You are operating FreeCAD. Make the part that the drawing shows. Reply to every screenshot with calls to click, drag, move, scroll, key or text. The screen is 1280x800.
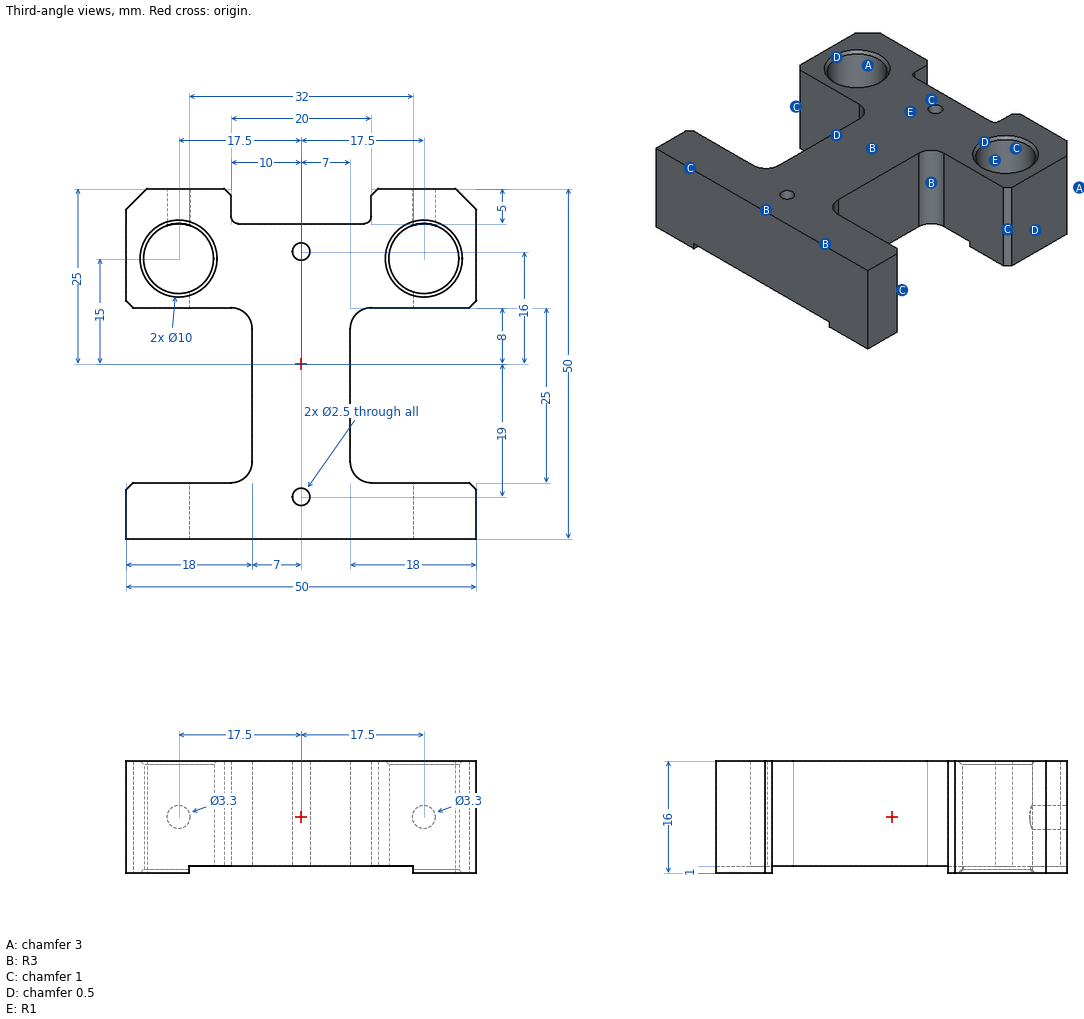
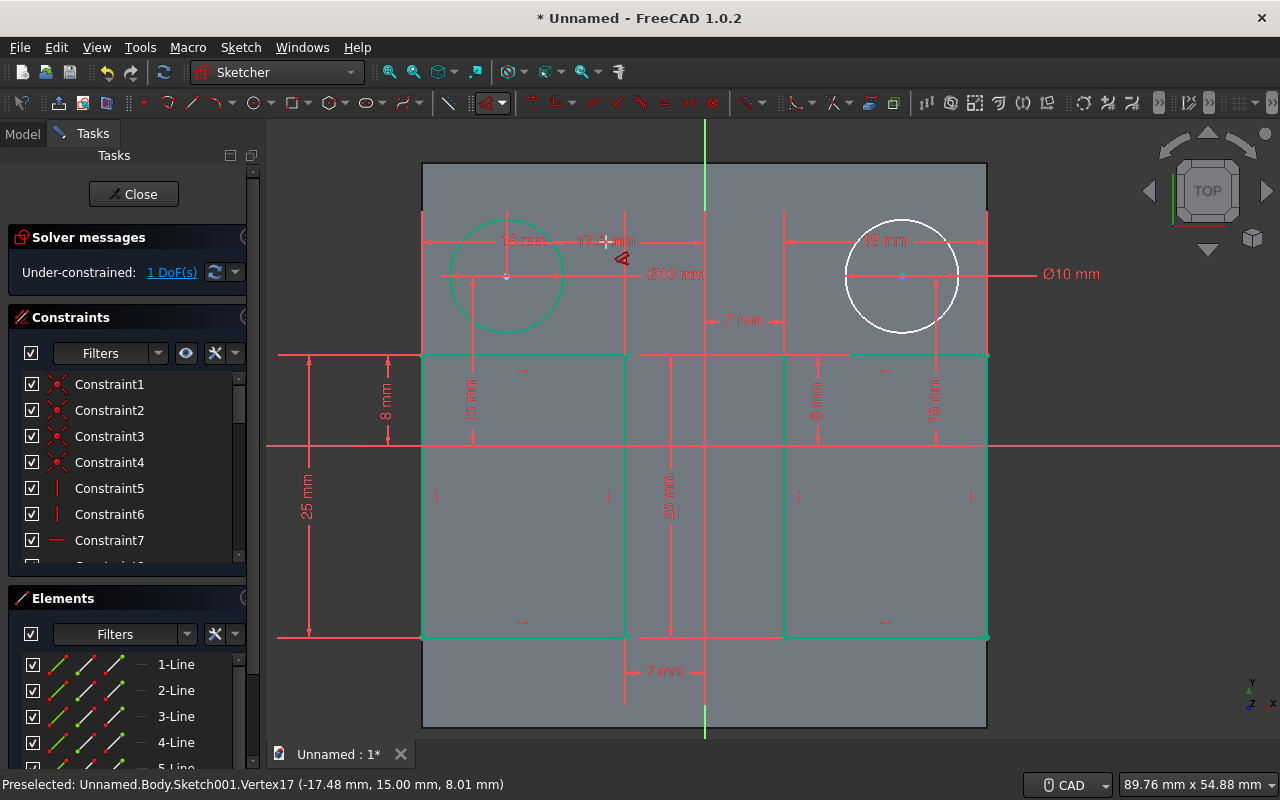
click(902, 276)
click(803, 242)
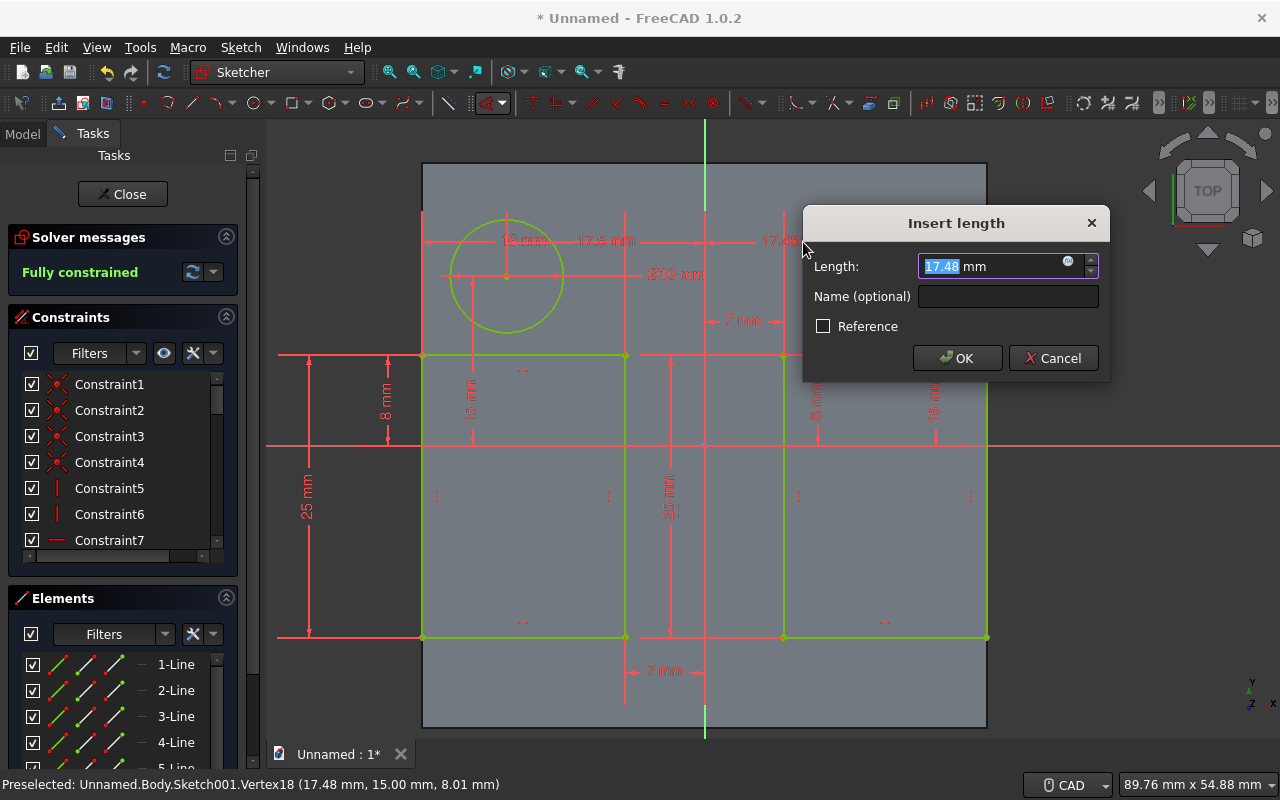
text(17.5)
key(Return)
key(Escape)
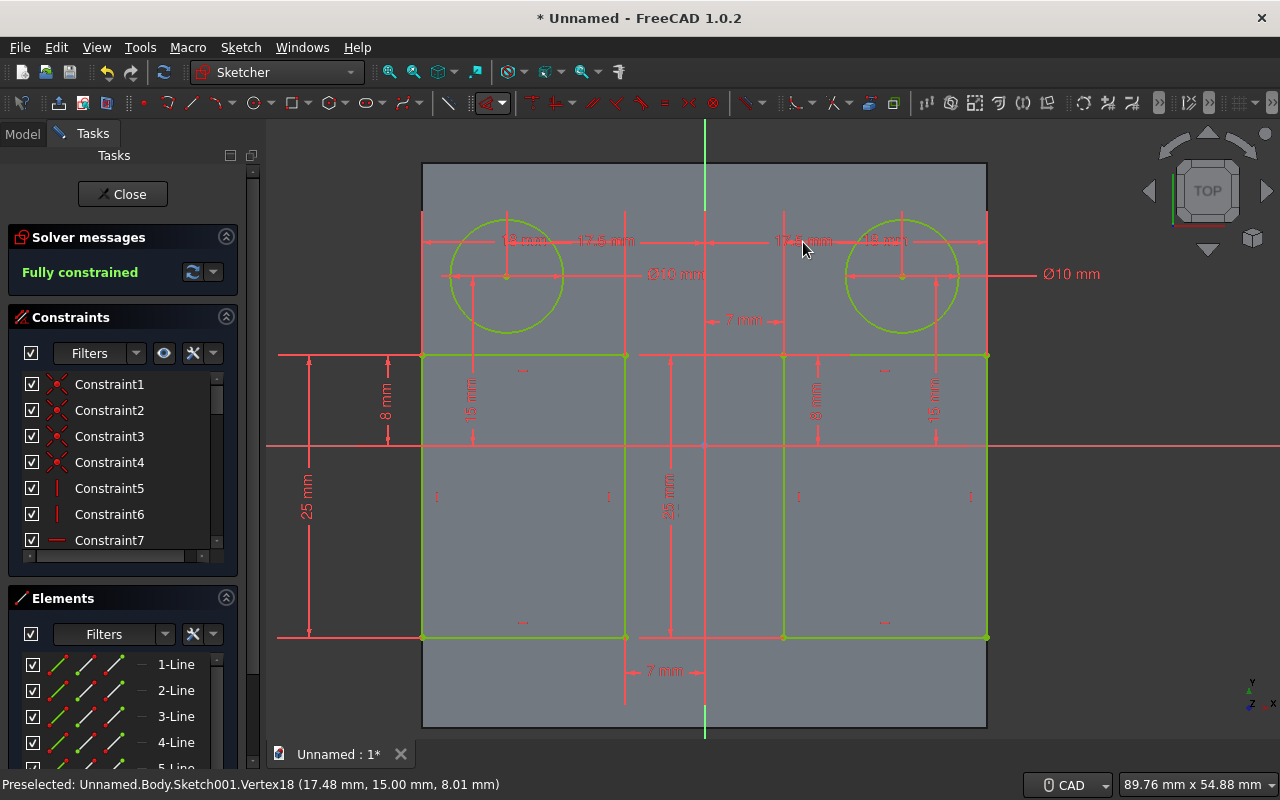
click(123, 194)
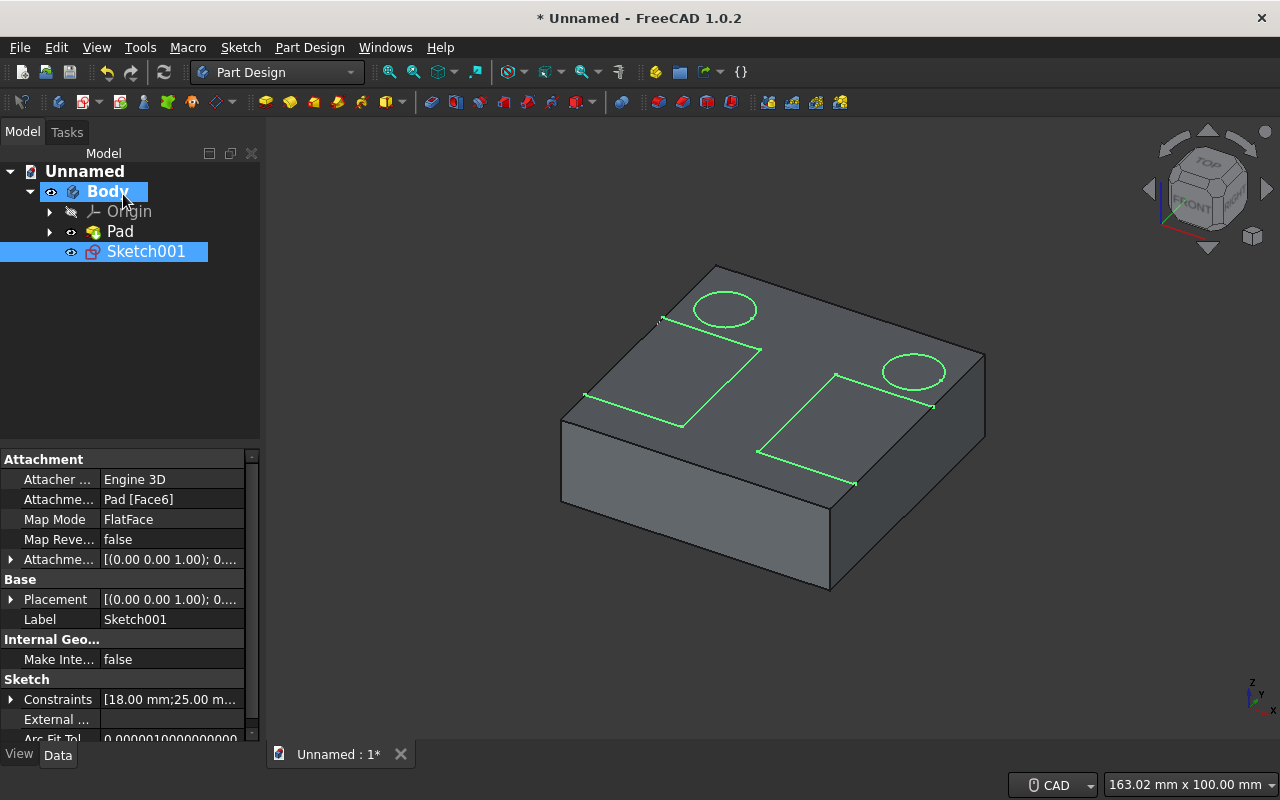
click(432, 102)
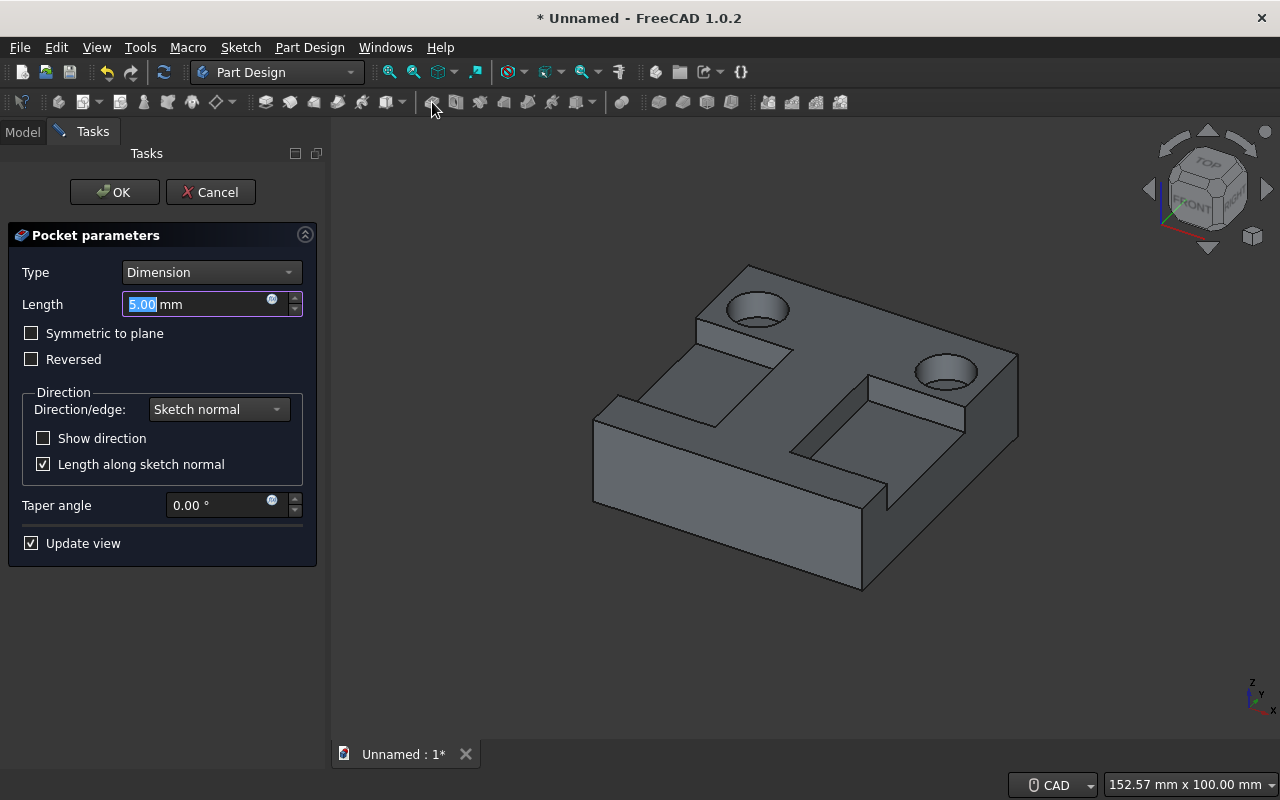
click(212, 272)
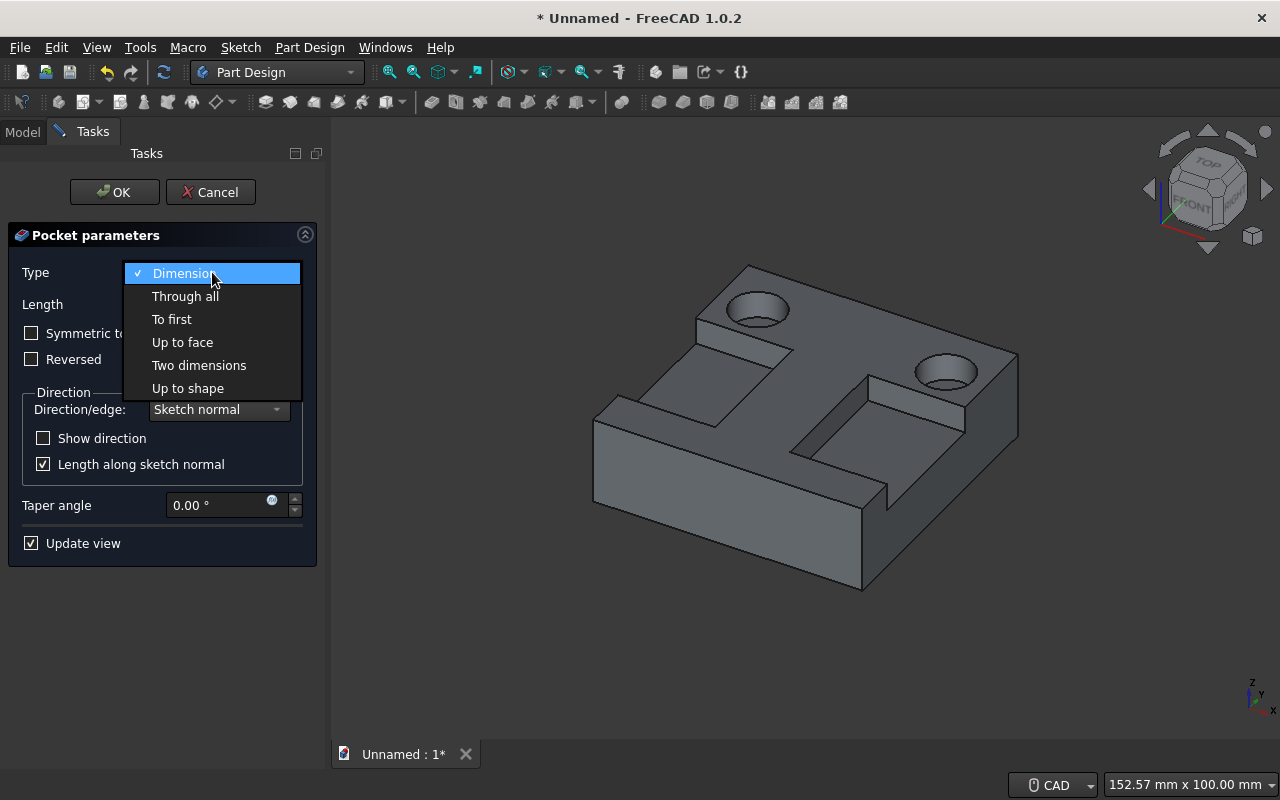
click(212, 296)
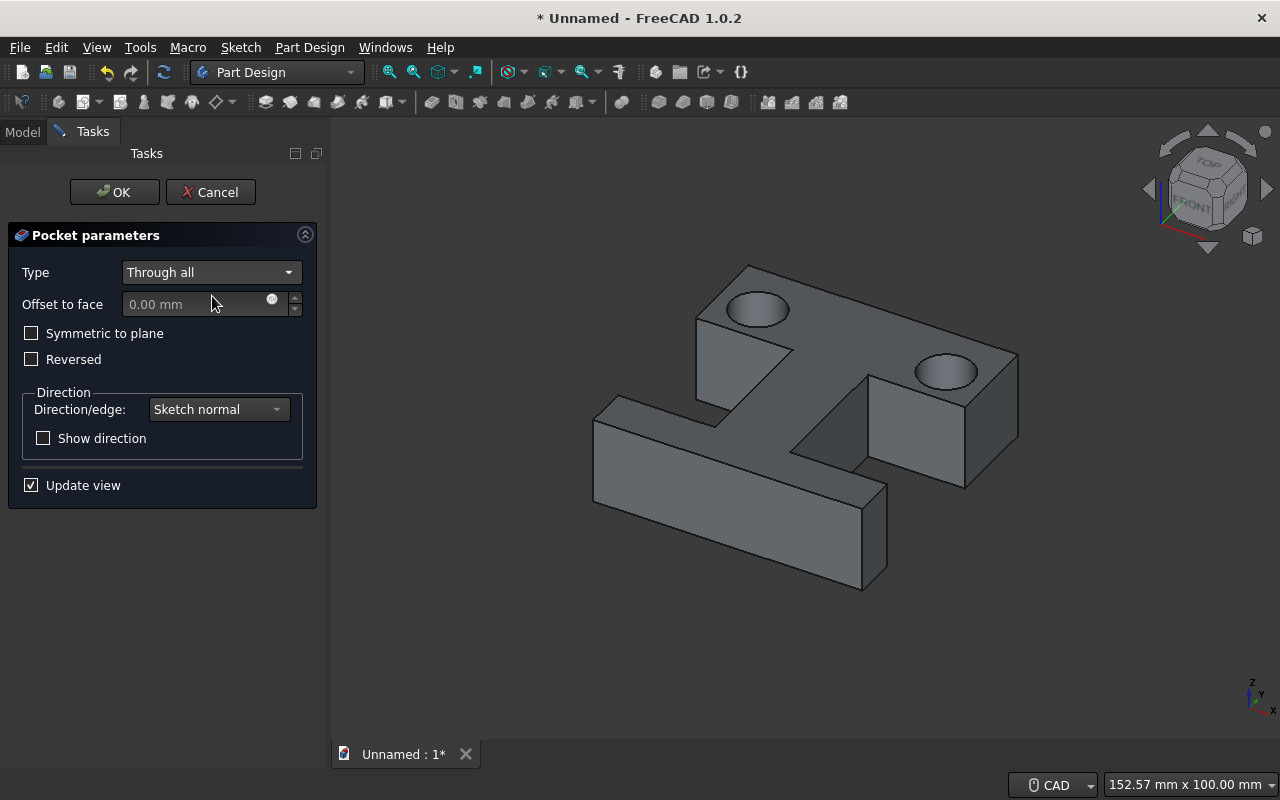
click(115, 192)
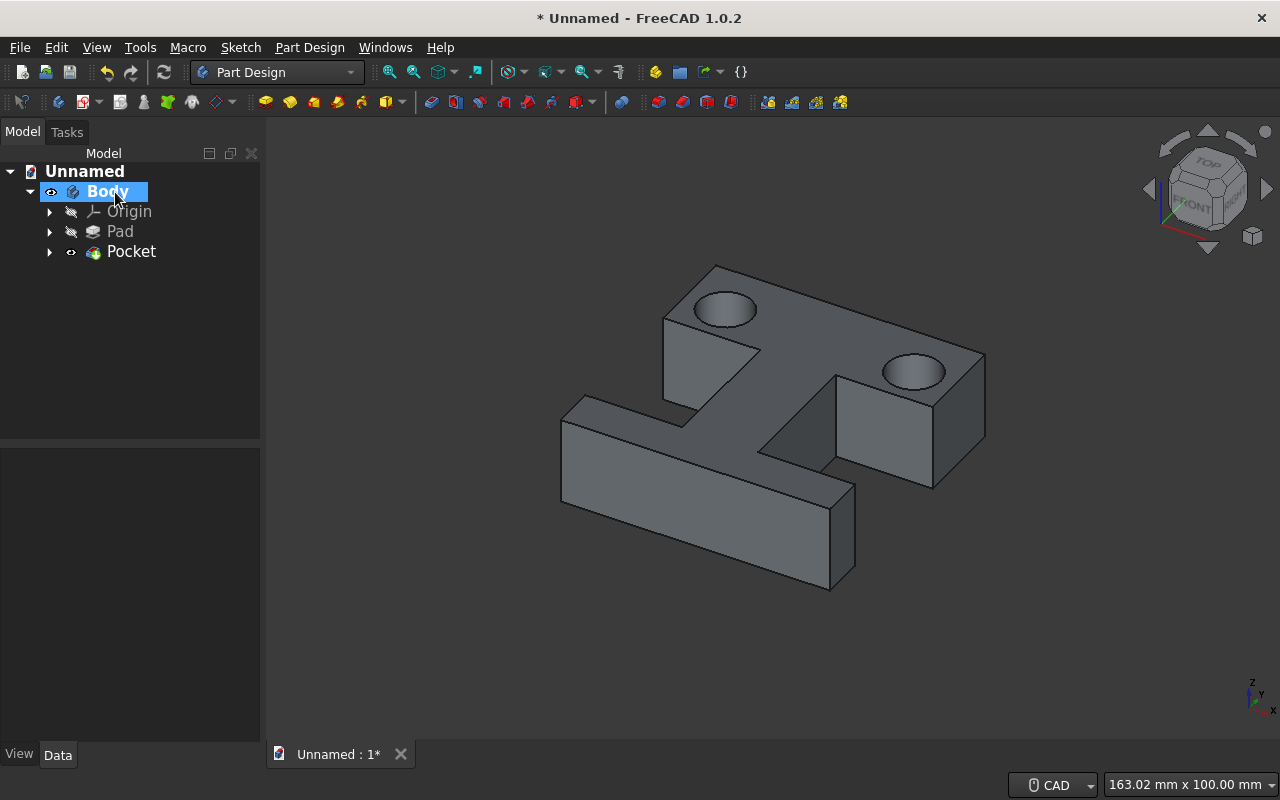
key(4)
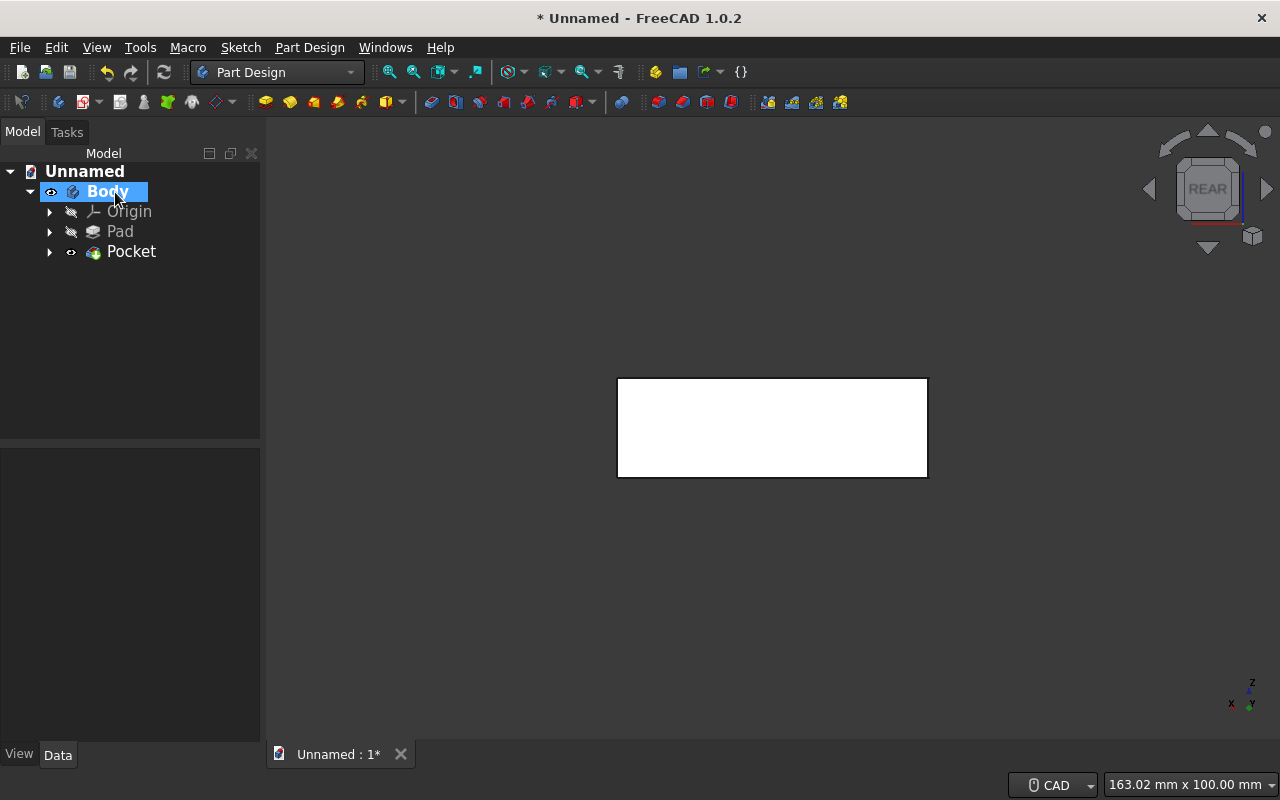
click(390, 72)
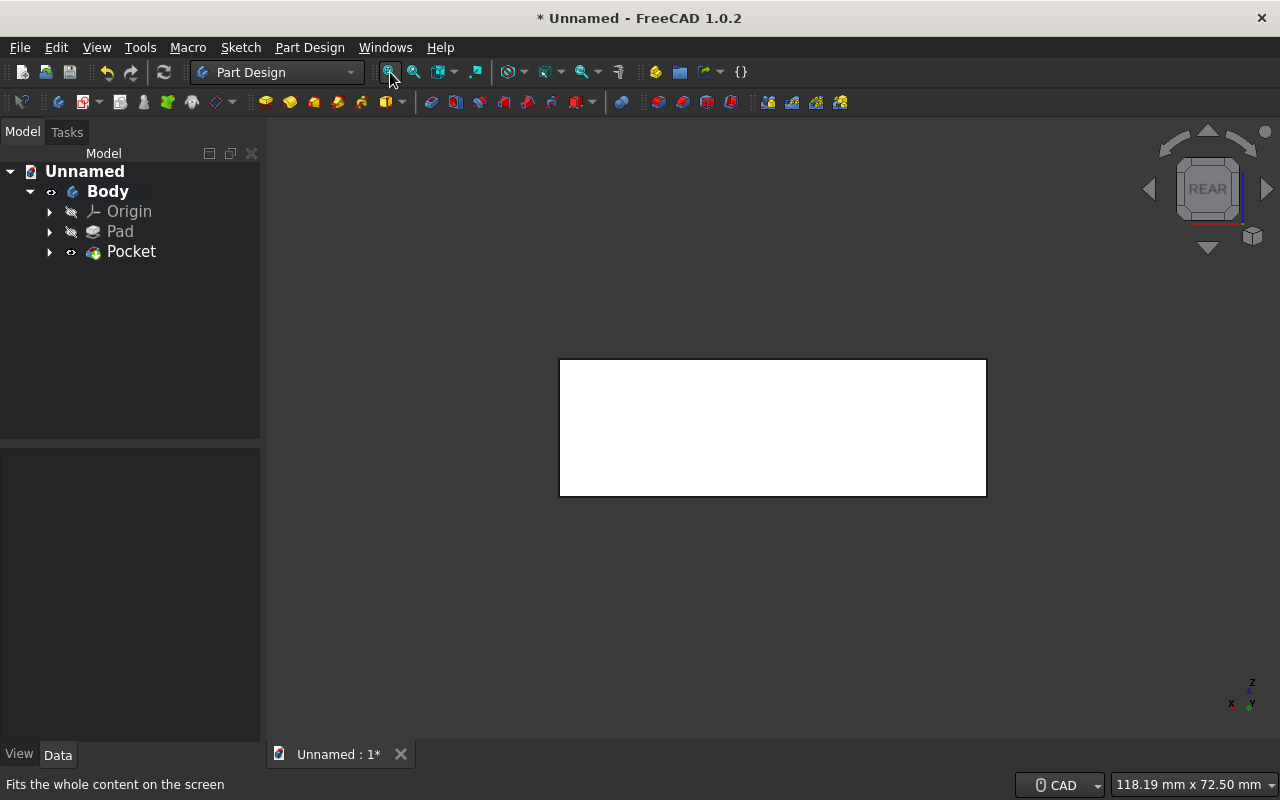
click(650, 427)